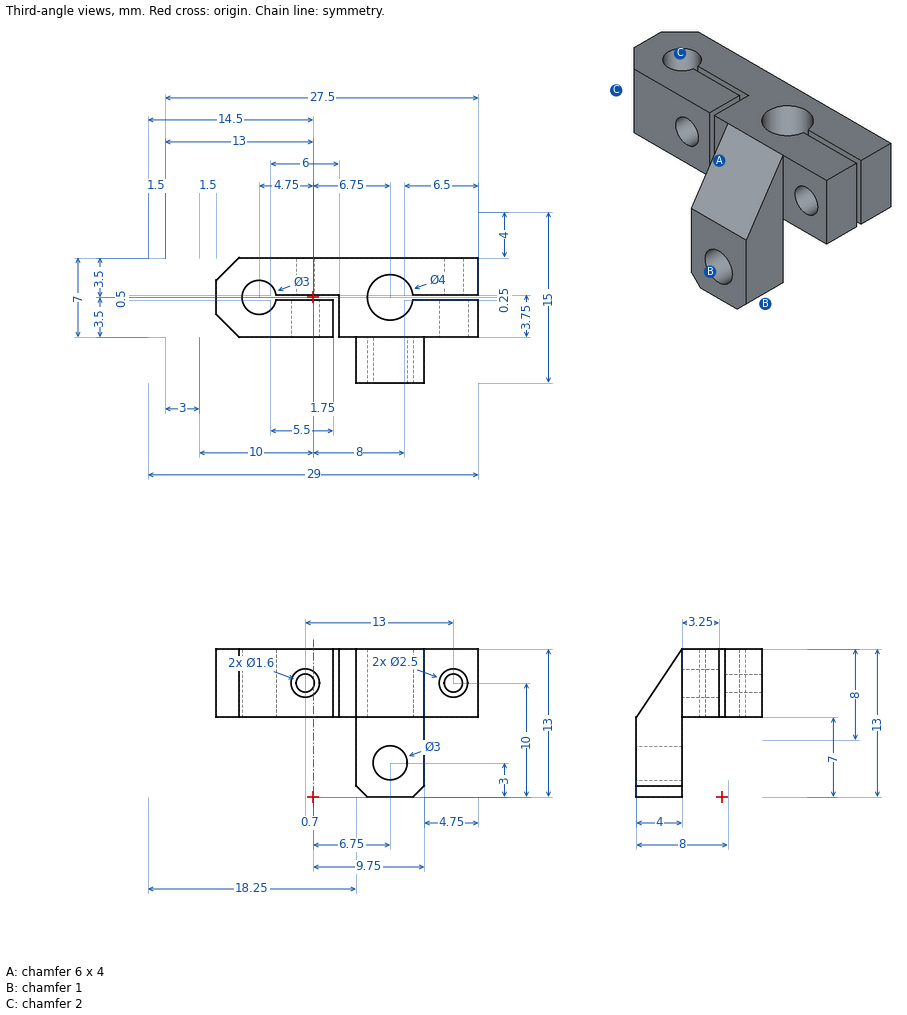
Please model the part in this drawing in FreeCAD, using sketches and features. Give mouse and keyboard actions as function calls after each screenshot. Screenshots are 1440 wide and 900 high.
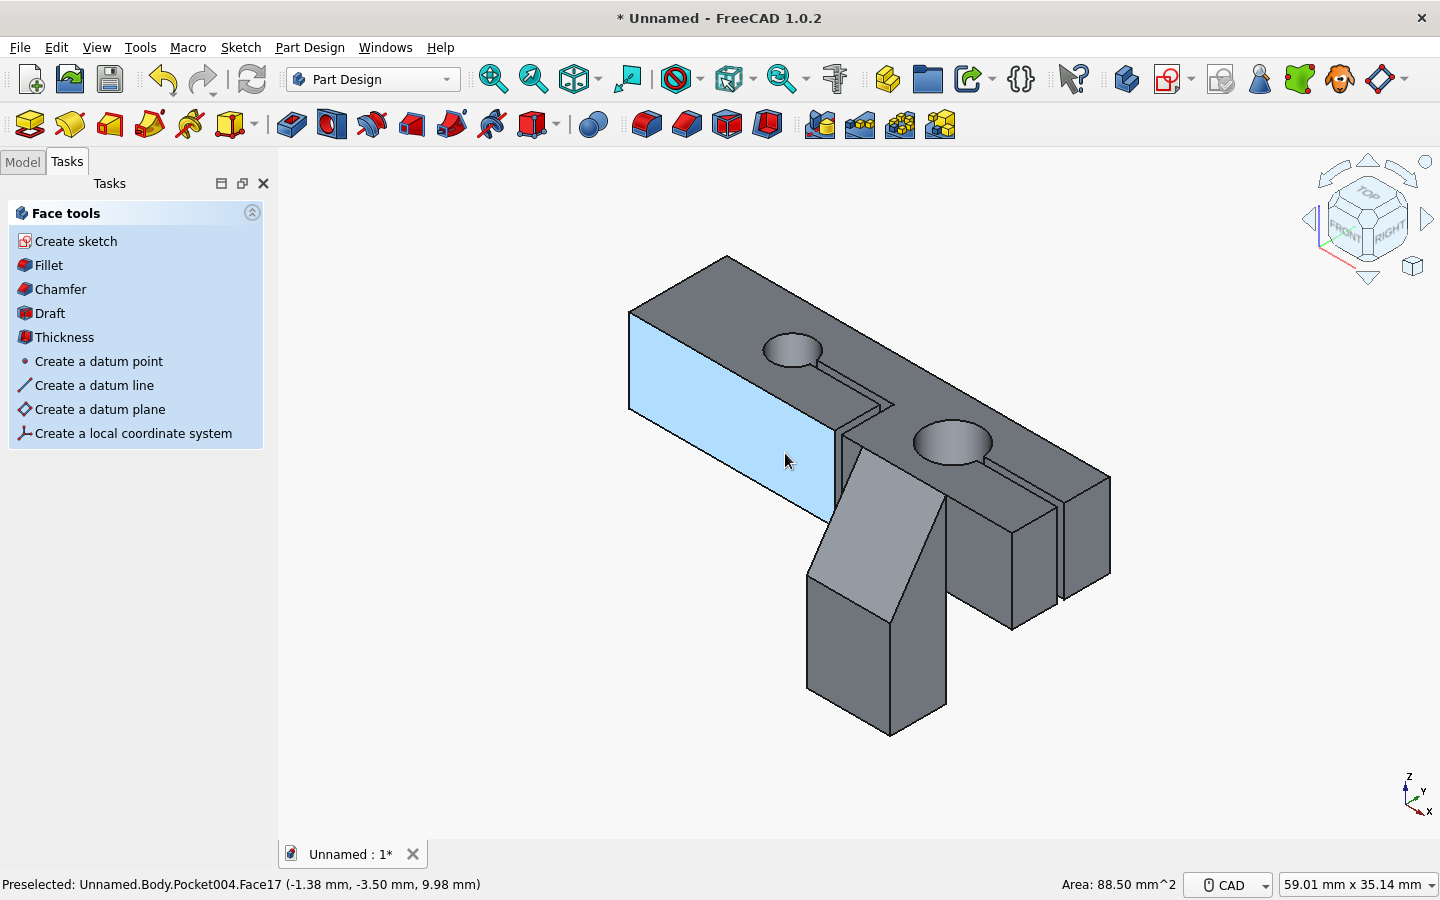
click(1168, 80)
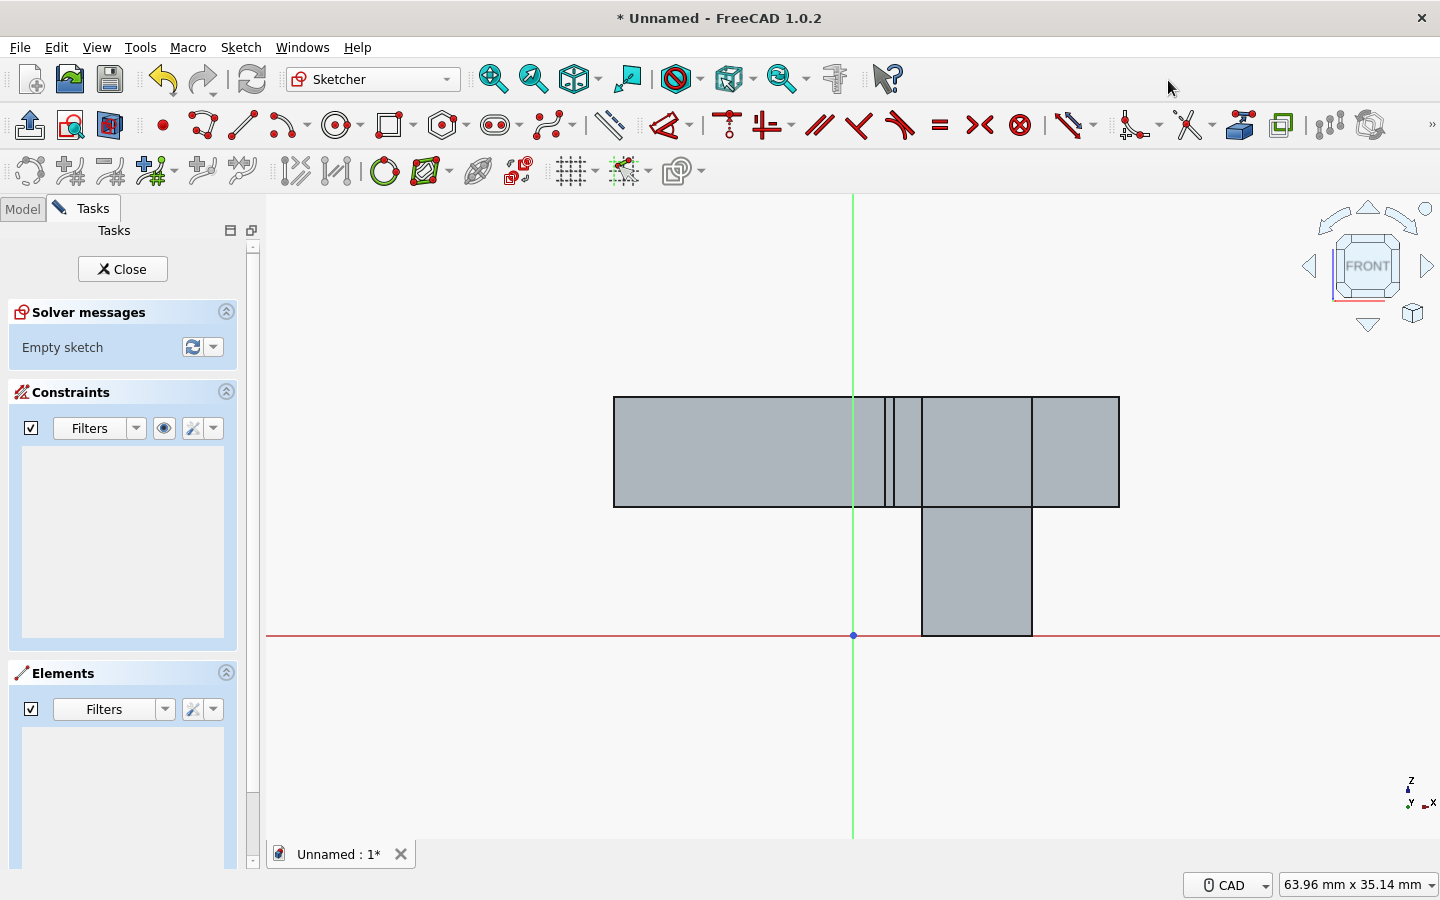
click(110, 126)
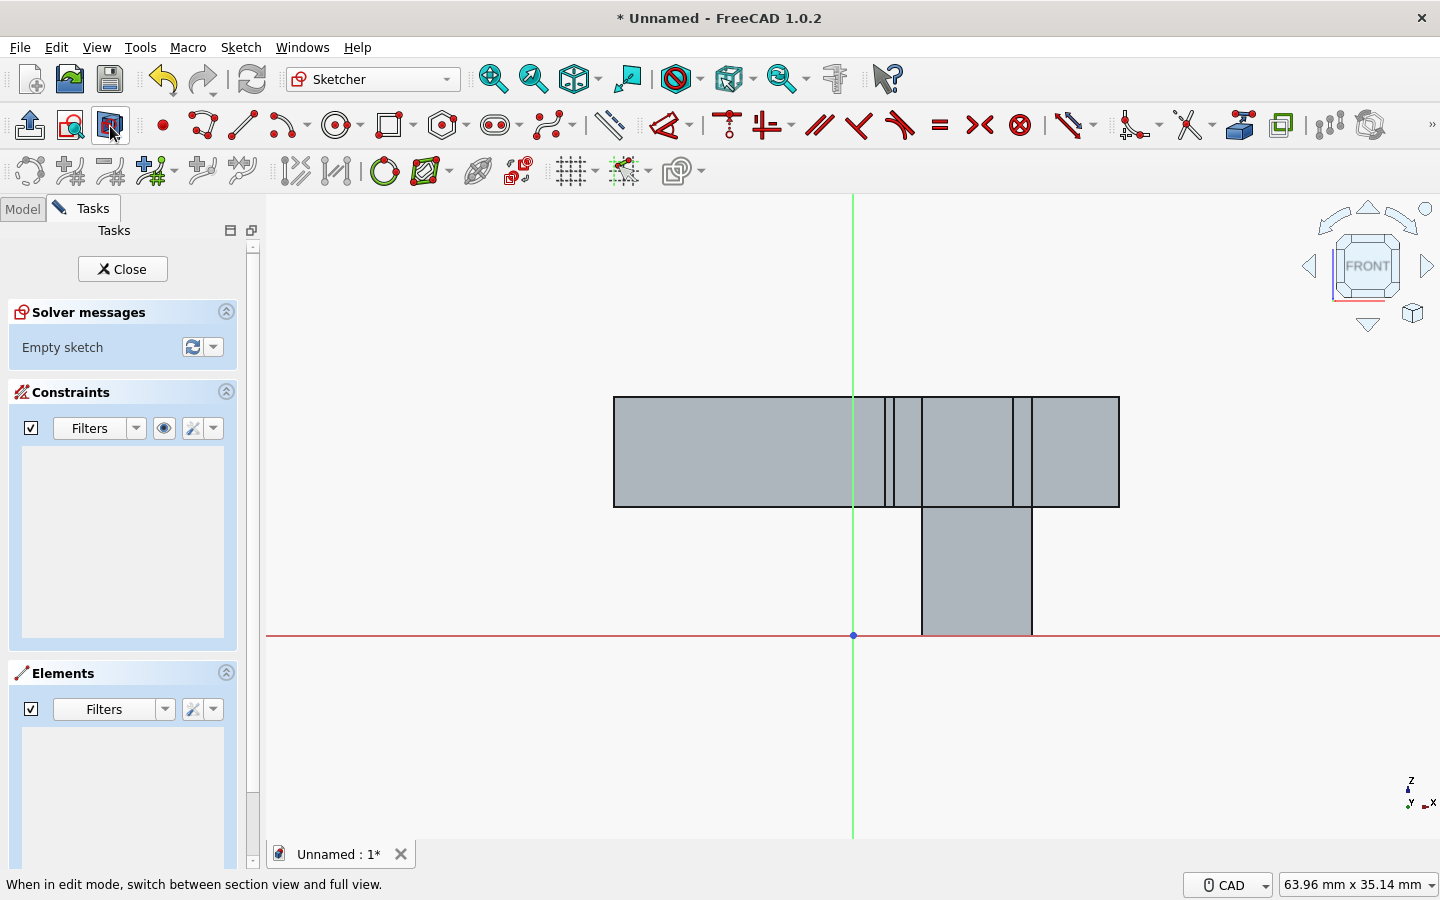
scroll(1172, 552, up, 3)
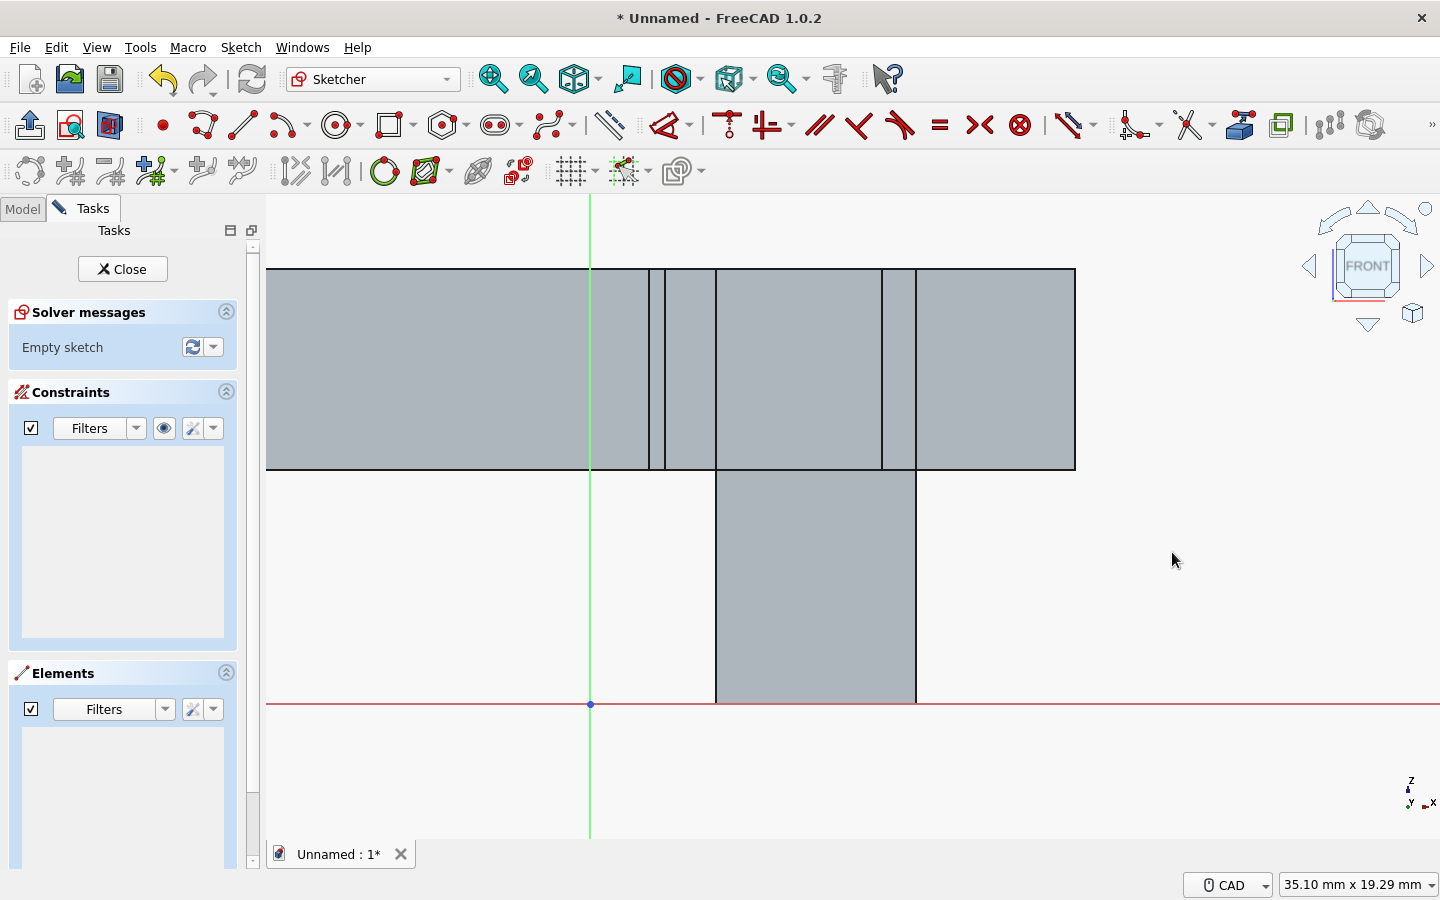
click(336, 126)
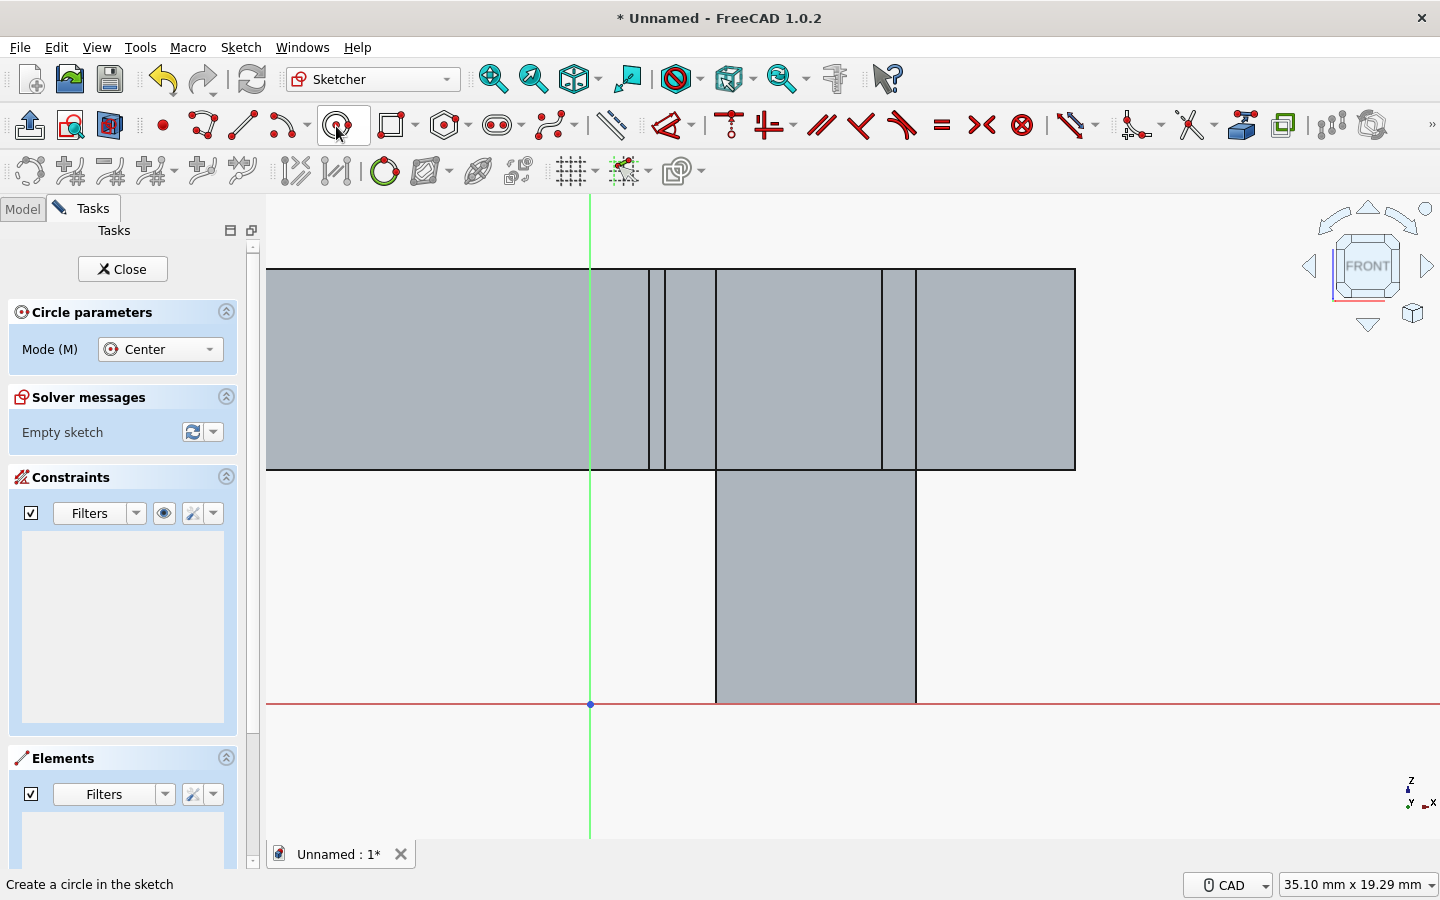
click(1001, 370)
move(1031, 340)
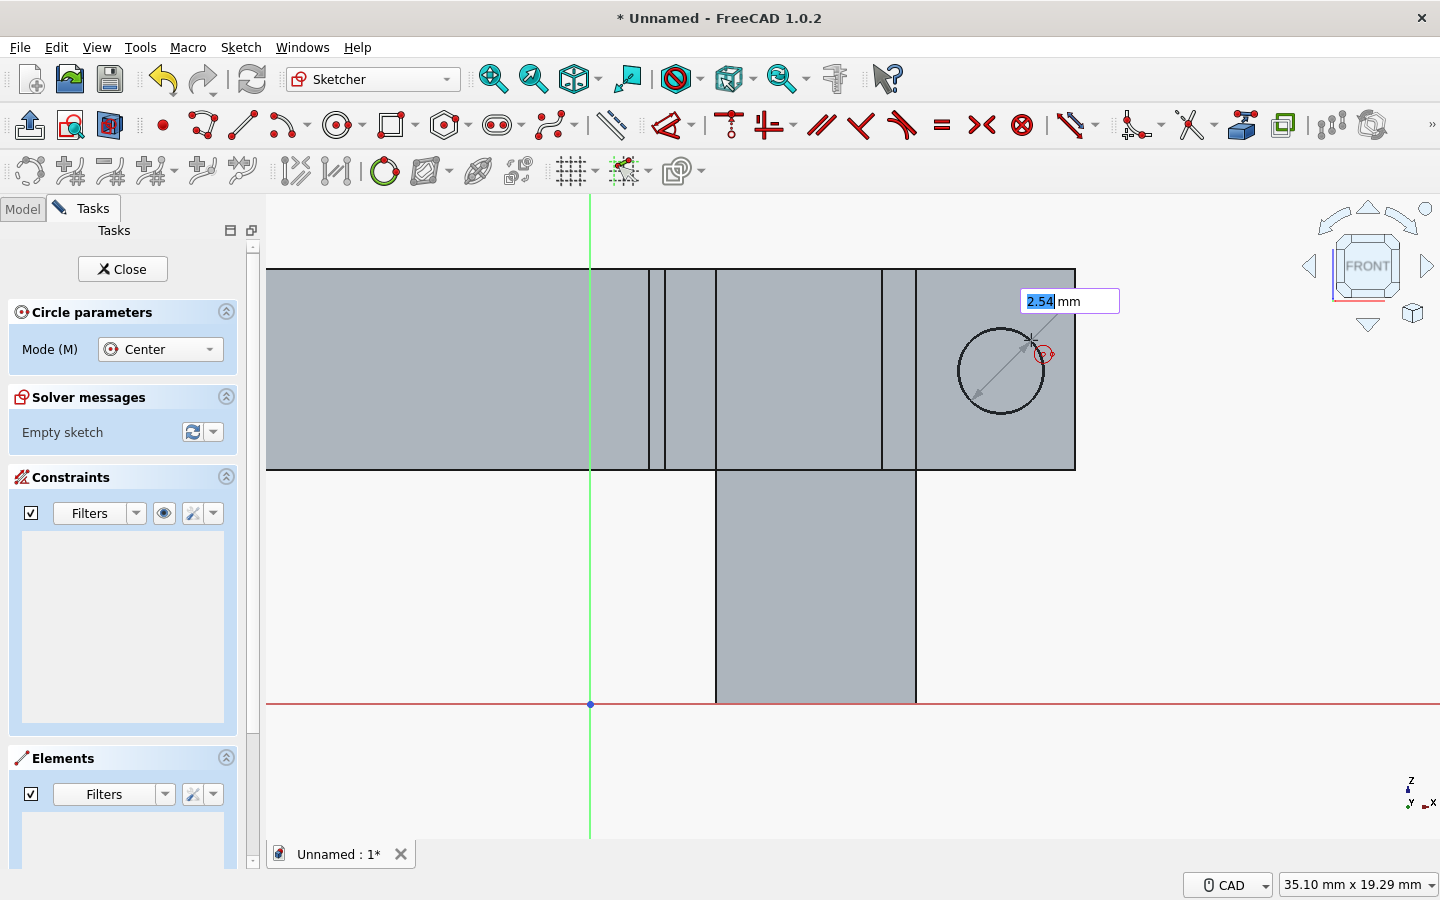
text(2.5)
key(Return)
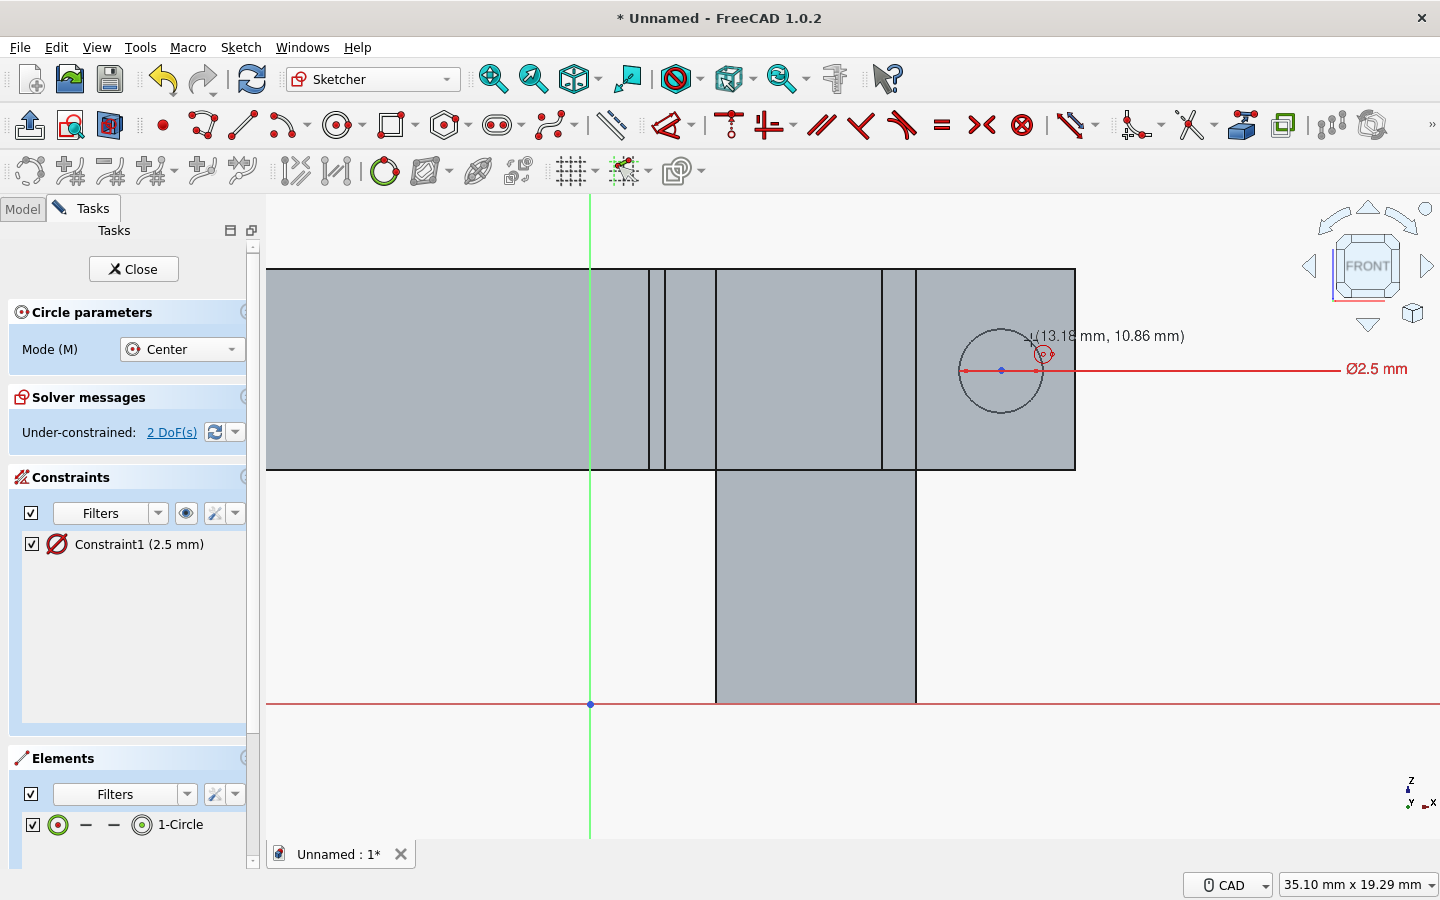
click(567, 370)
move(537, 340)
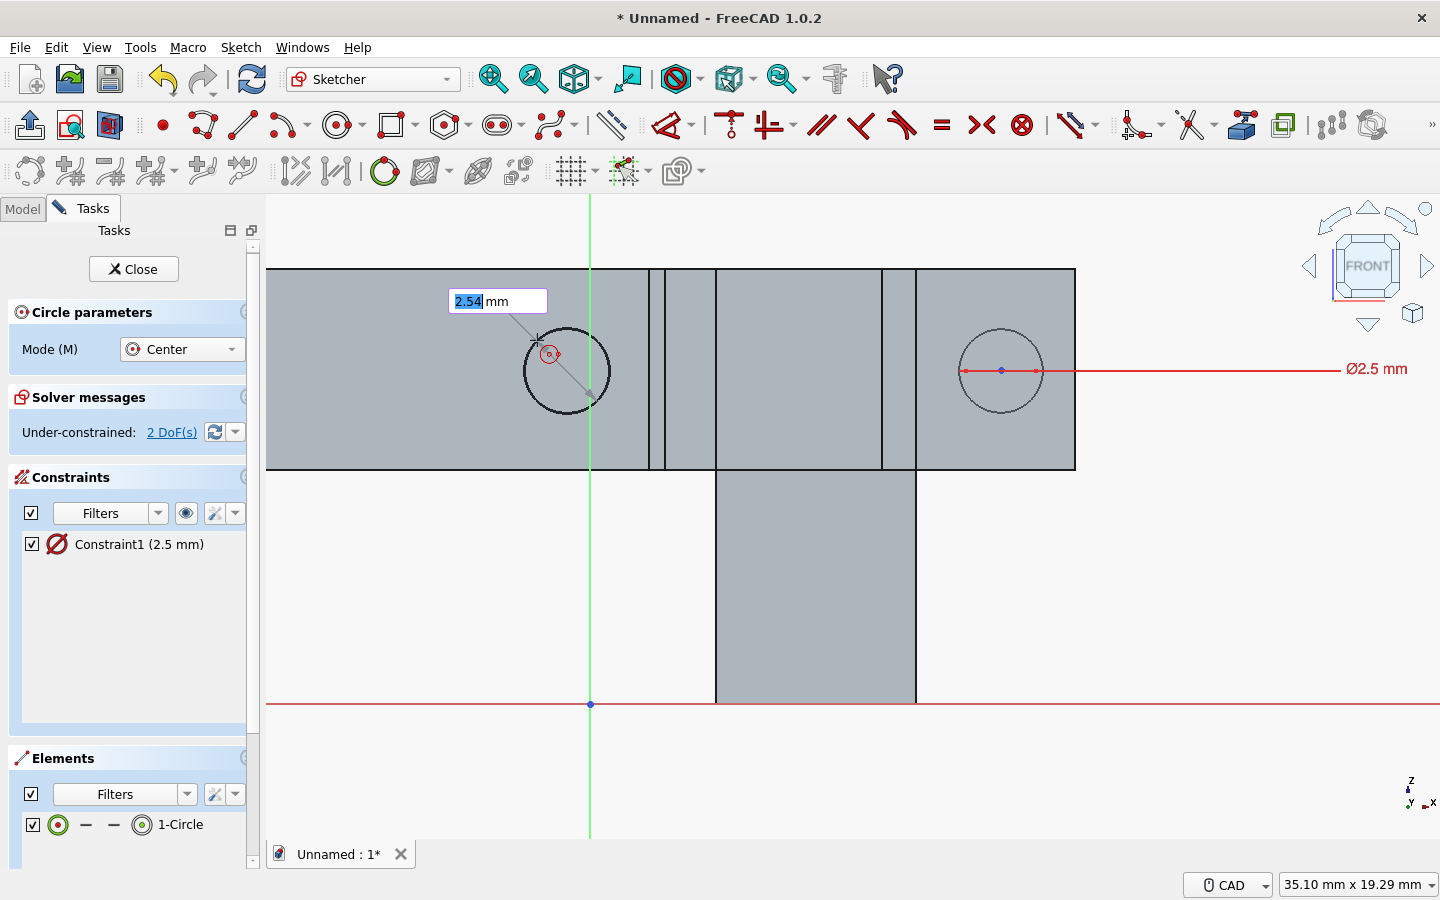
text(2.5)
key(Return)
key(Escape)